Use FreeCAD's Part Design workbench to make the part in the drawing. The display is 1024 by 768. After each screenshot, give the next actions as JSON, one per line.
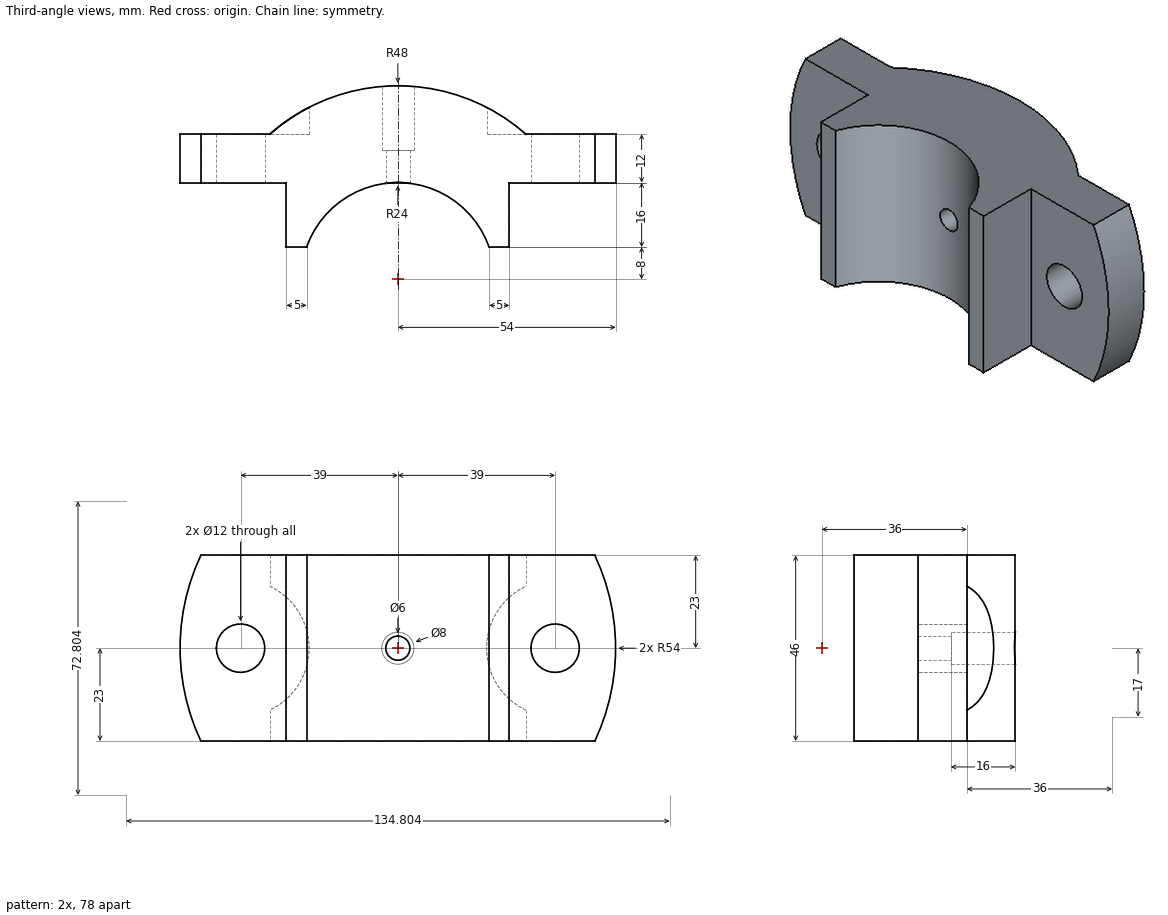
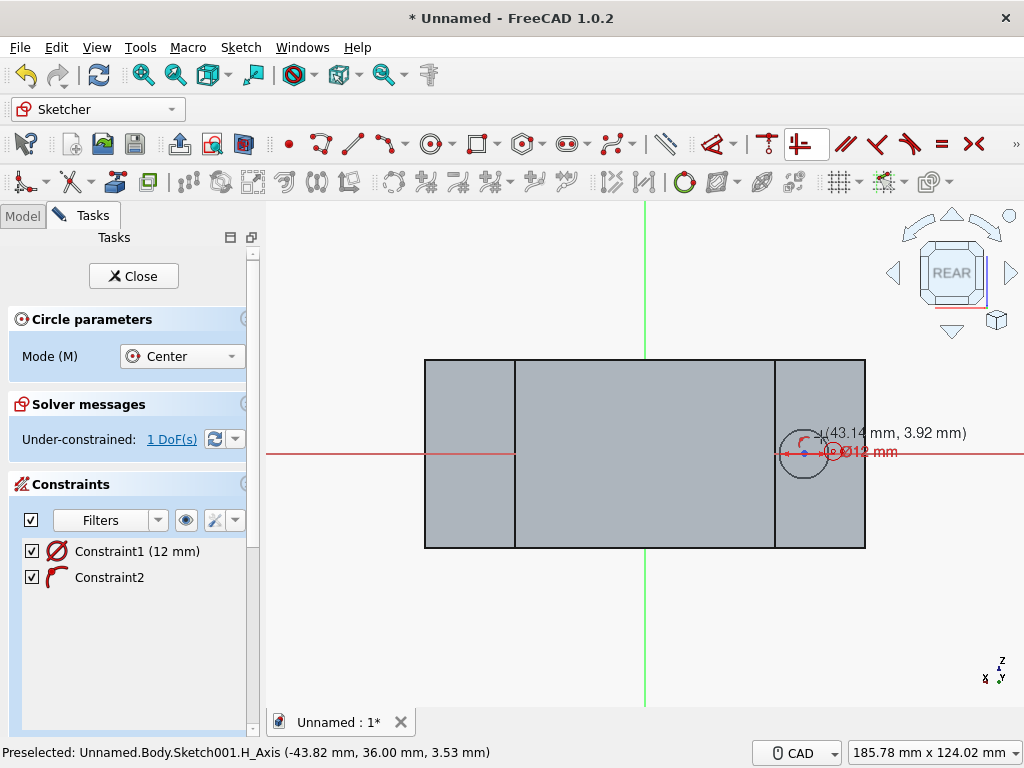
{"action": "left_click", "coordinate": [486, 454]}
{"action": "mouse_move", "coordinate": [503, 437]}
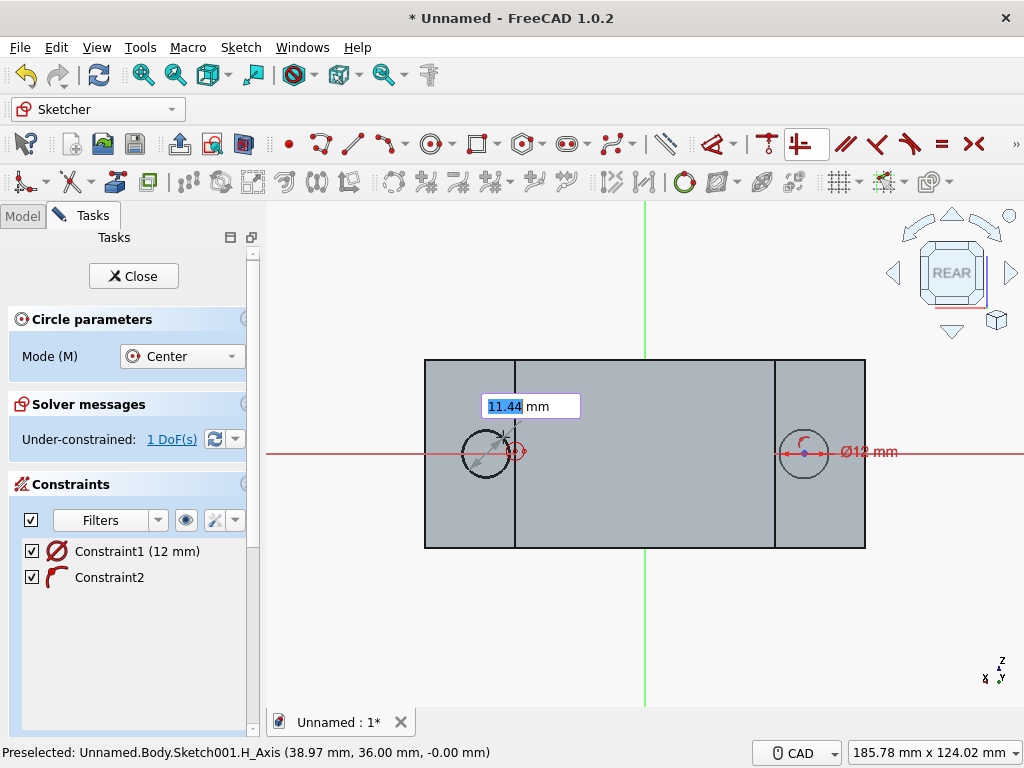
{"action": "type", "text": "12"}
{"action": "key", "text": "Return"}
{"action": "key", "text": "Escape"}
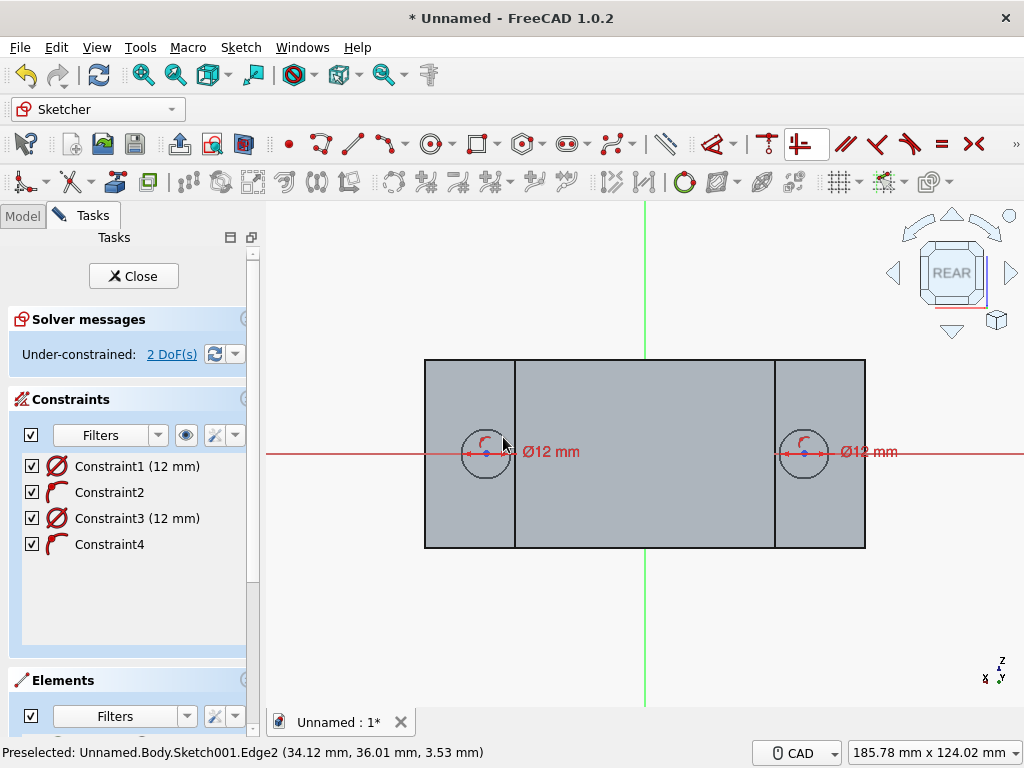
{"action": "left_click", "coordinate": [712, 144]}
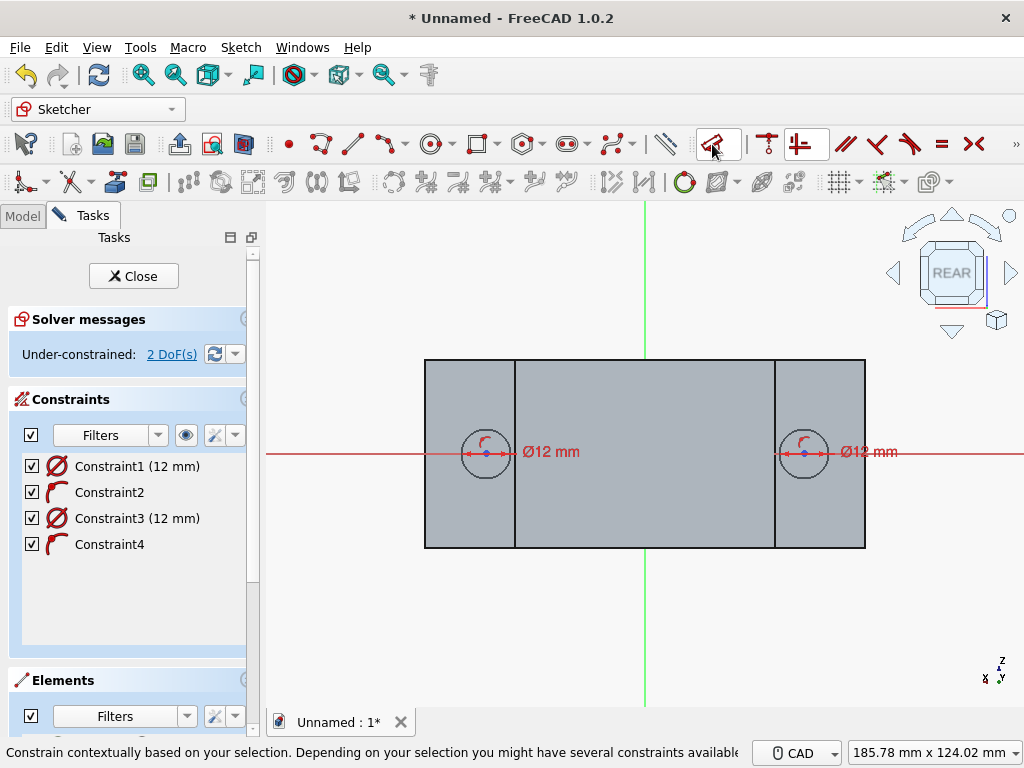
{"action": "left_click", "coordinate": [804, 454]}
{"action": "left_click", "coordinate": [724, 488]}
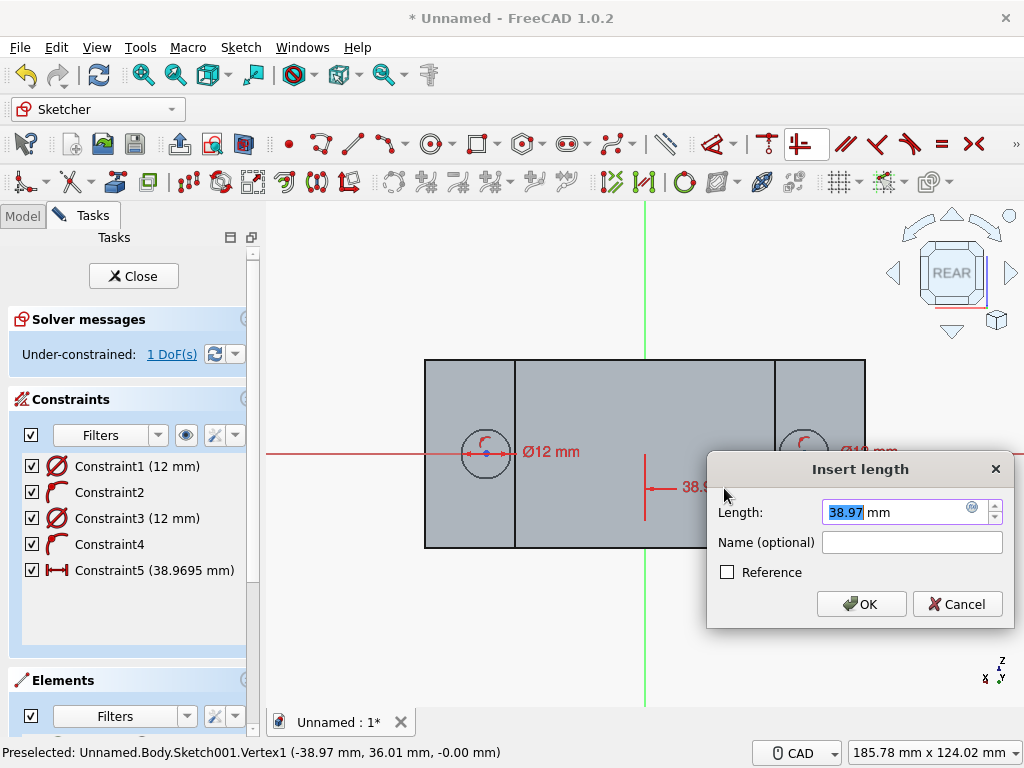
{"action": "type", "text": "39"}
{"action": "key", "text": "Return"}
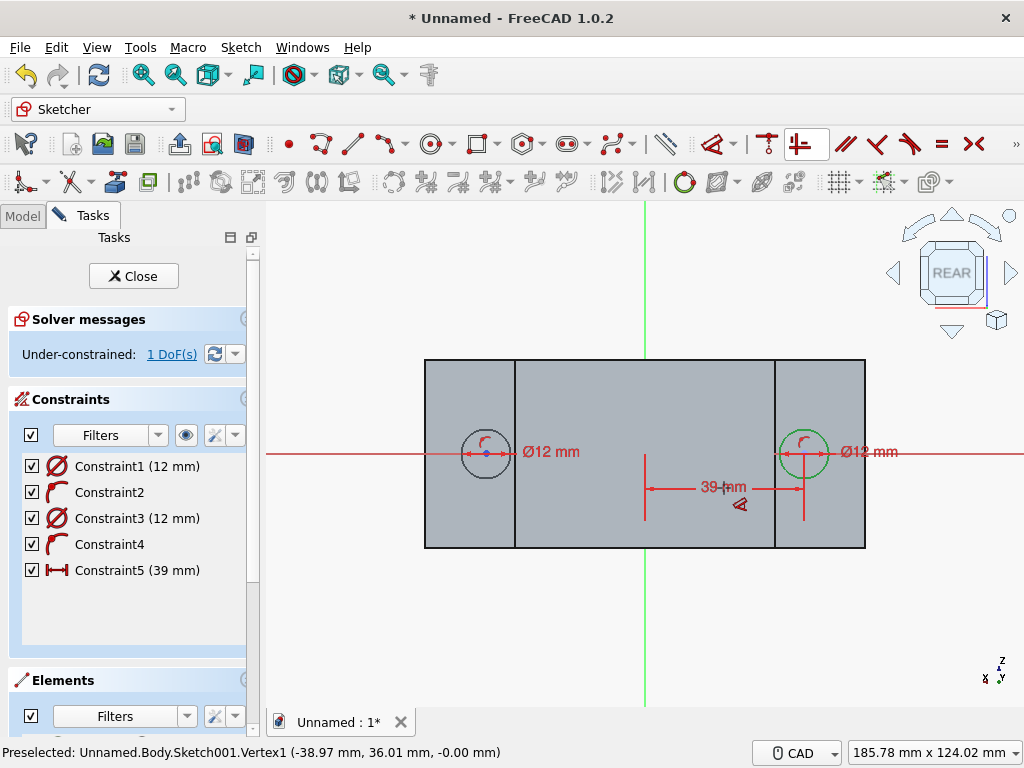
{"action": "left_click", "coordinate": [486, 454]}
{"action": "left_click", "coordinate": [565, 488]}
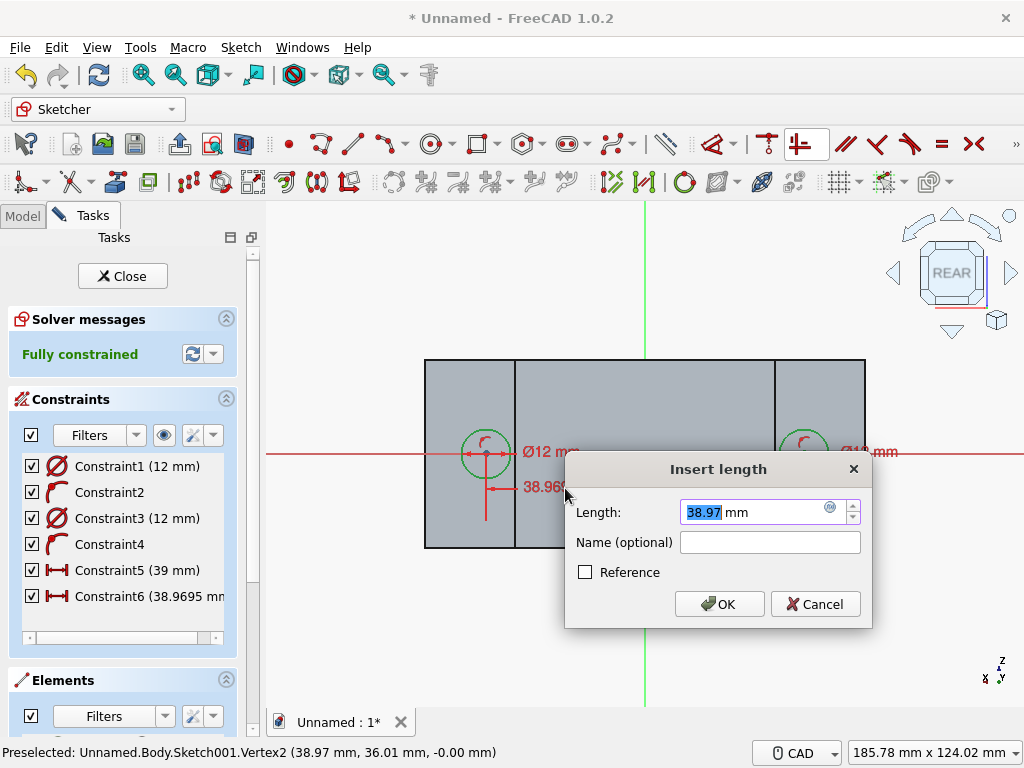
{"action": "type", "text": "39"}
{"action": "key", "text": "Return"}
{"action": "key", "text": "Escape"}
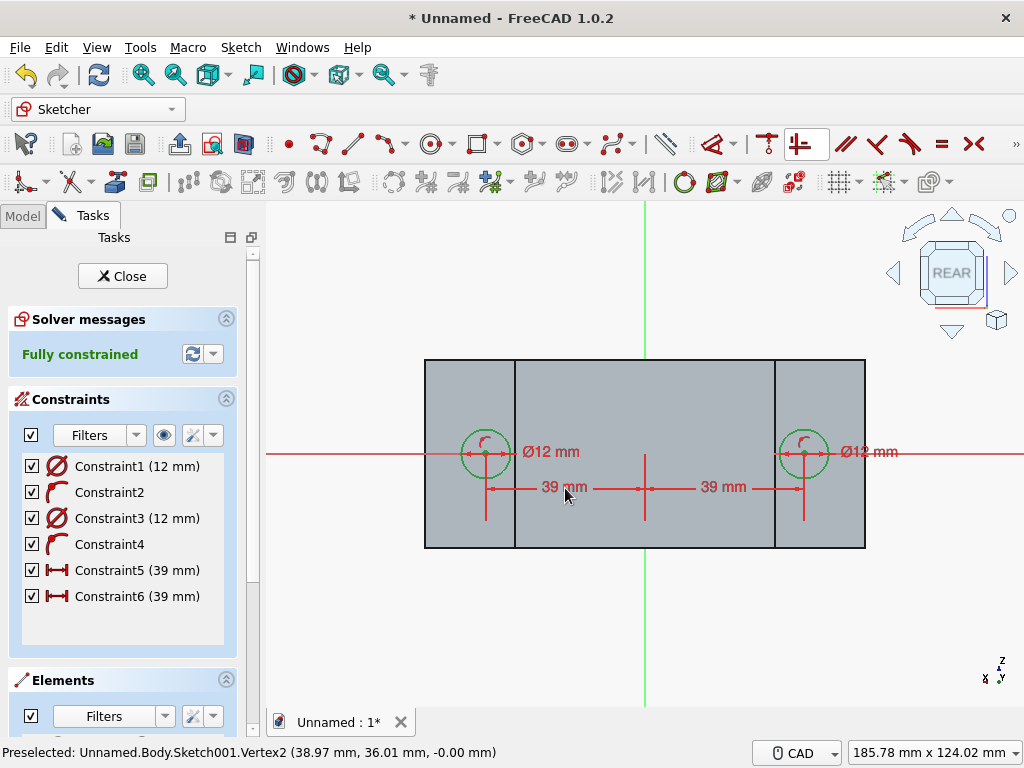
{"action": "left_click", "coordinate": [123, 276]}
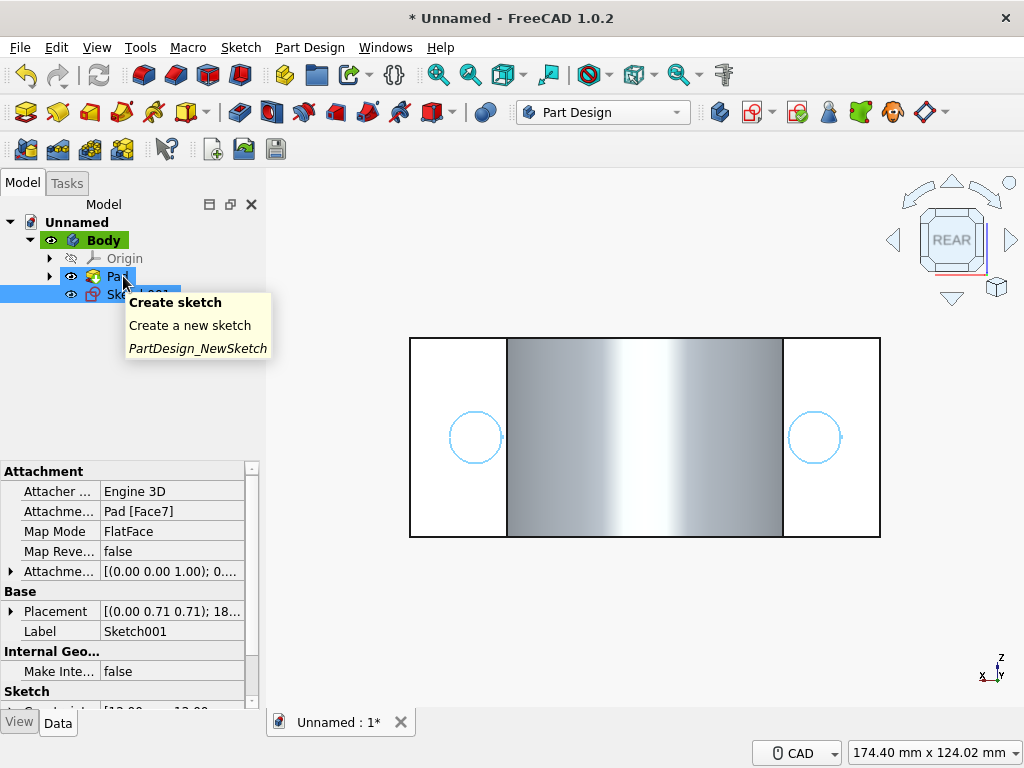
{"action": "left_click", "coordinate": [272, 112]}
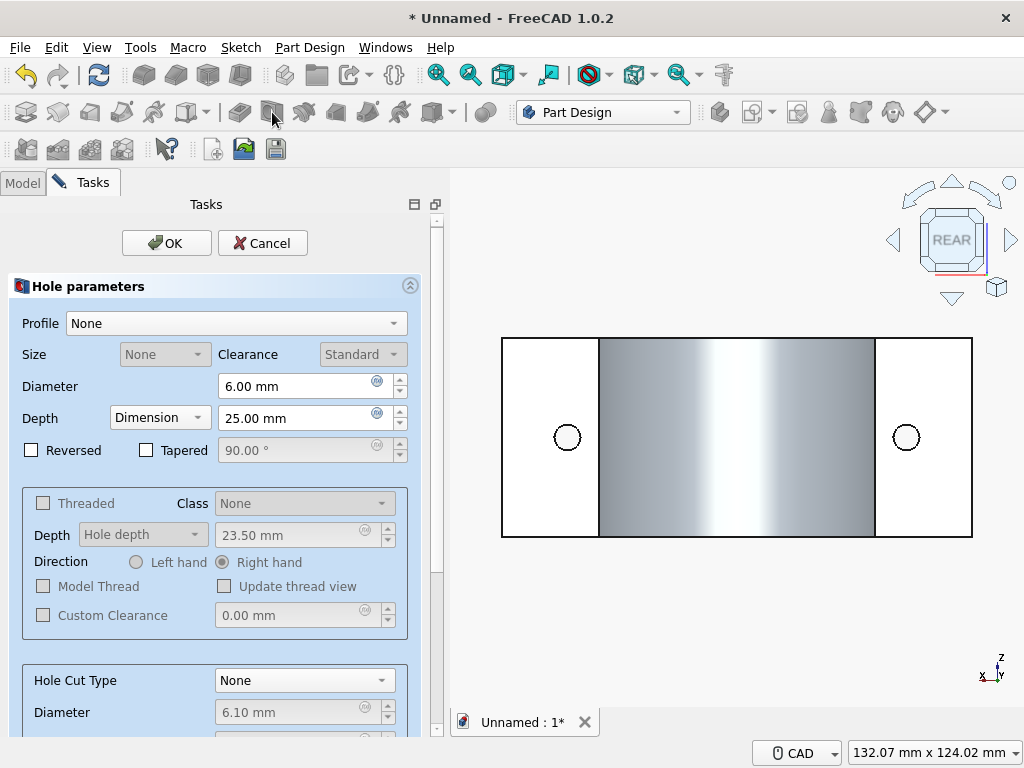
{"action": "triple_click", "coordinate": [305, 386]}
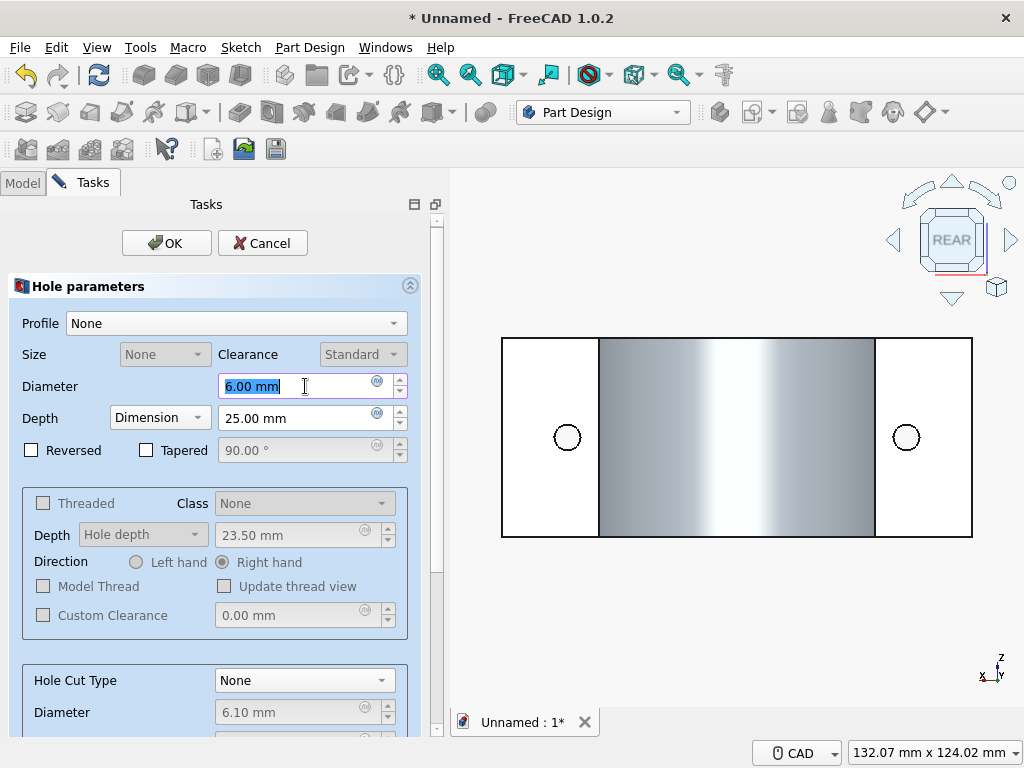
{"action": "type", "text": "12"}
{"action": "key", "text": "Tab"}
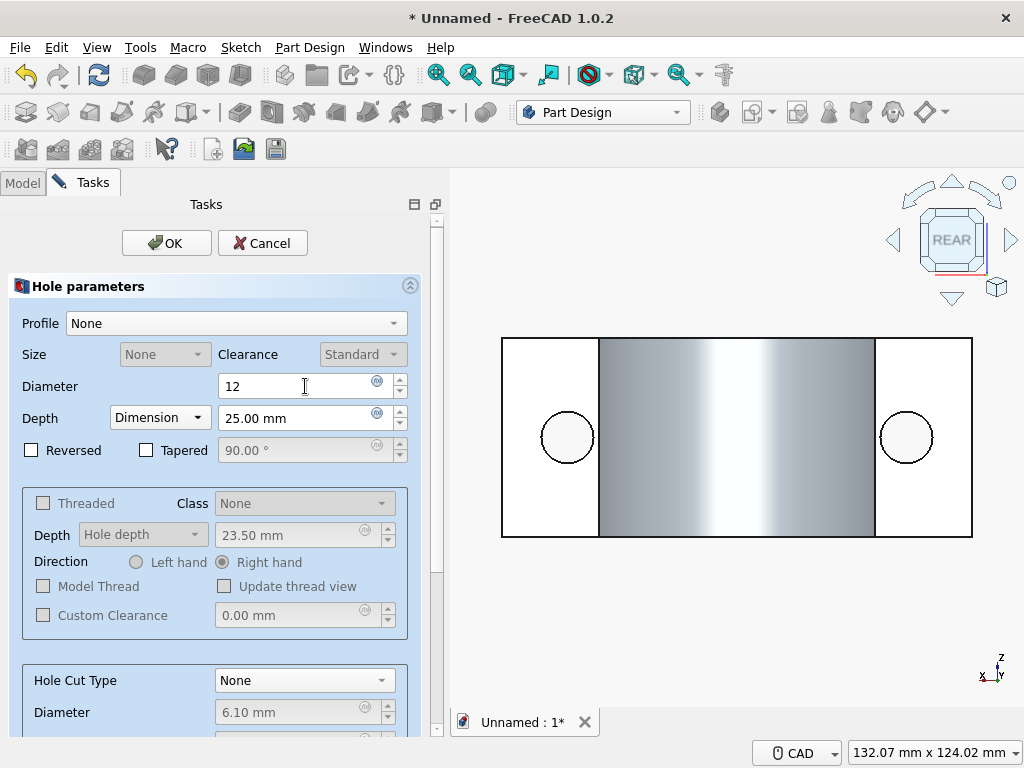
{"action": "left_click", "coordinate": [161, 418]}